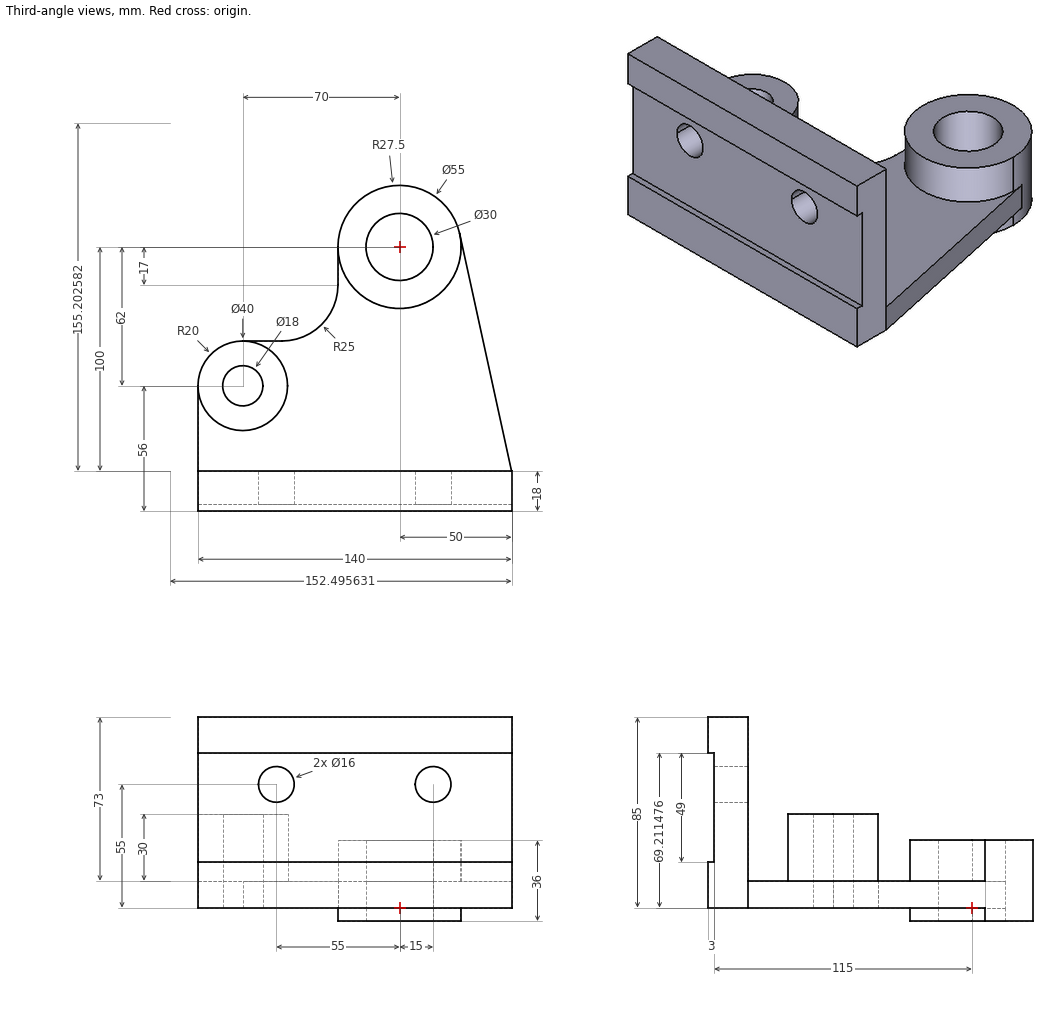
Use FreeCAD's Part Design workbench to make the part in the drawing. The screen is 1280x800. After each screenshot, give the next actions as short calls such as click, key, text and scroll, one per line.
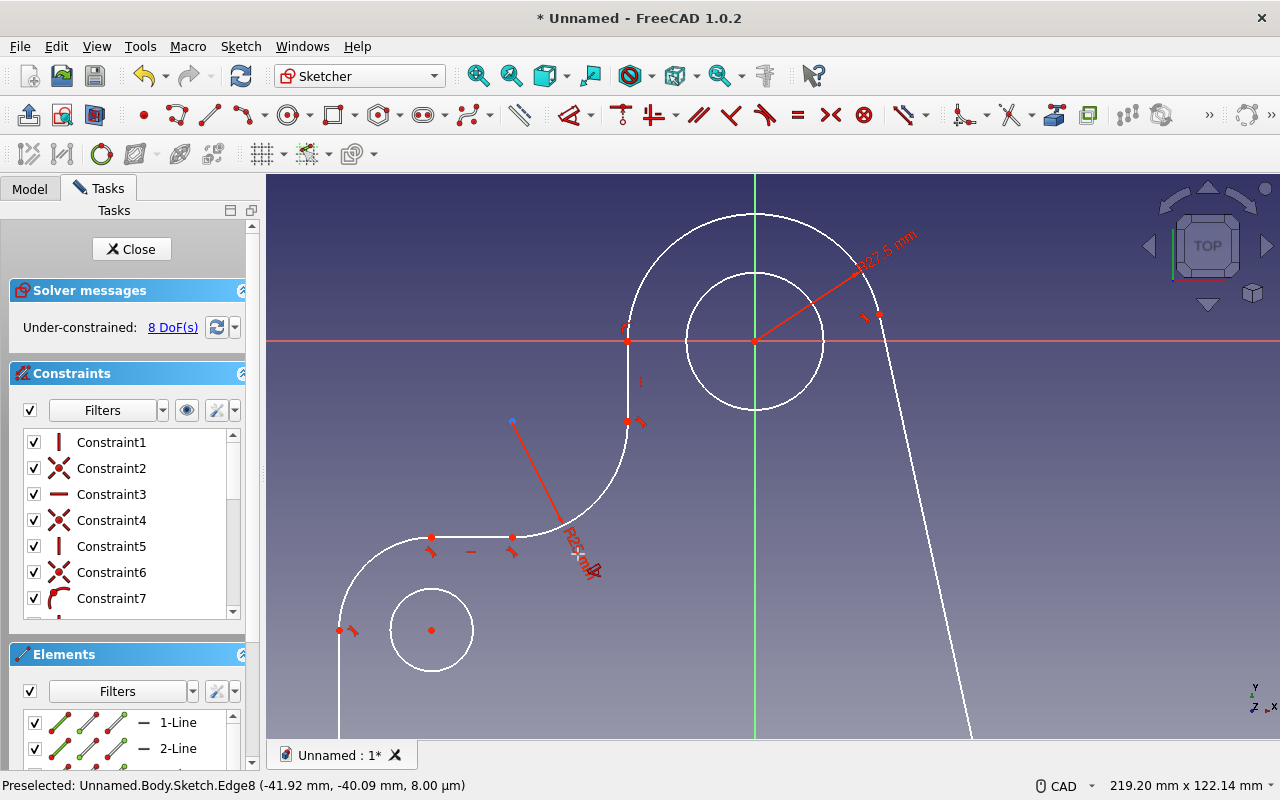
click(390, 548)
click(376, 519)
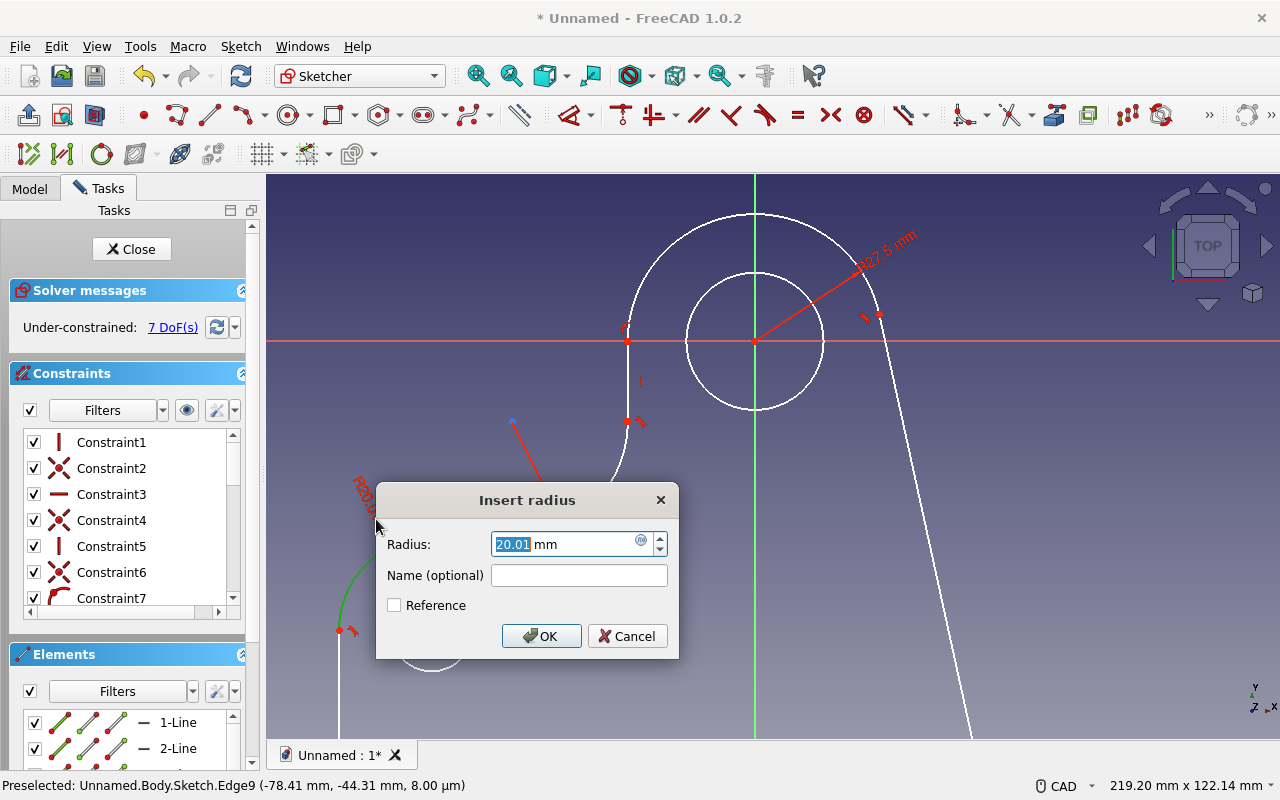
text(20)
key(Return)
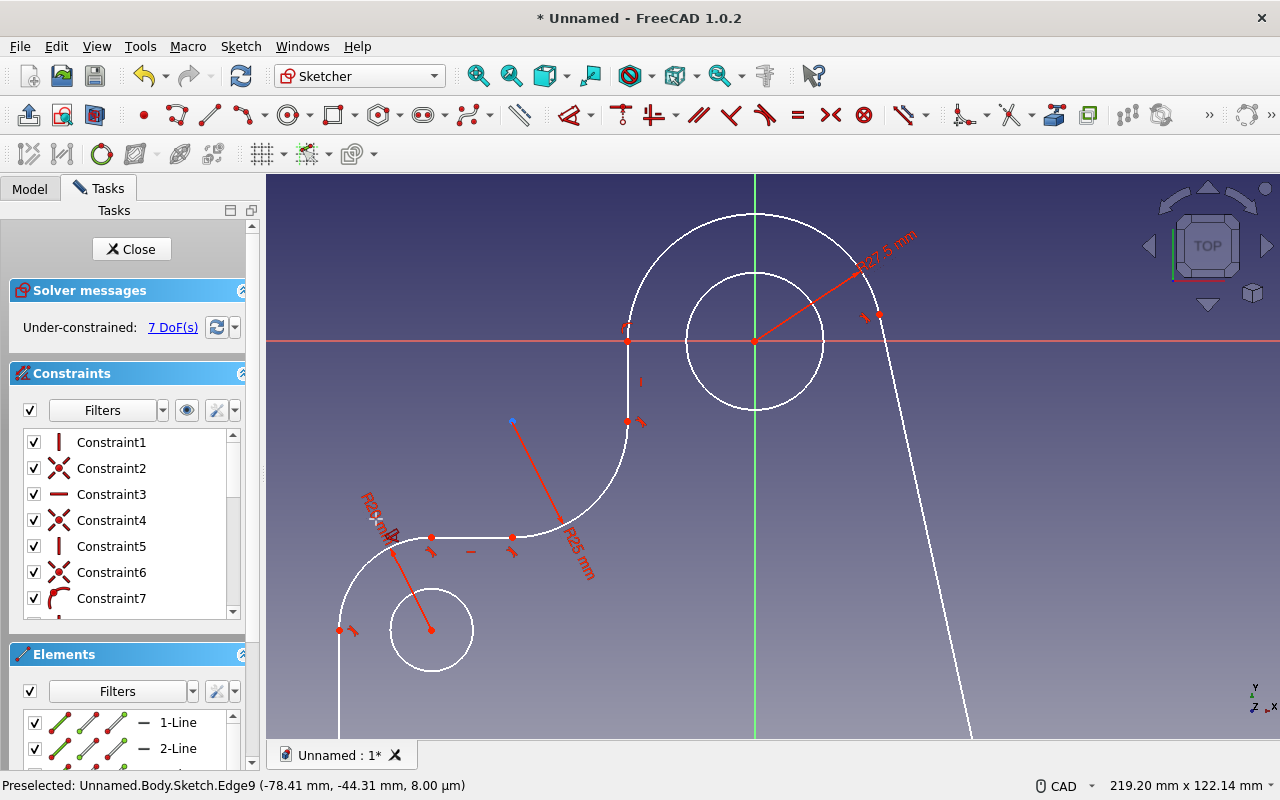
click(461, 601)
click(484, 578)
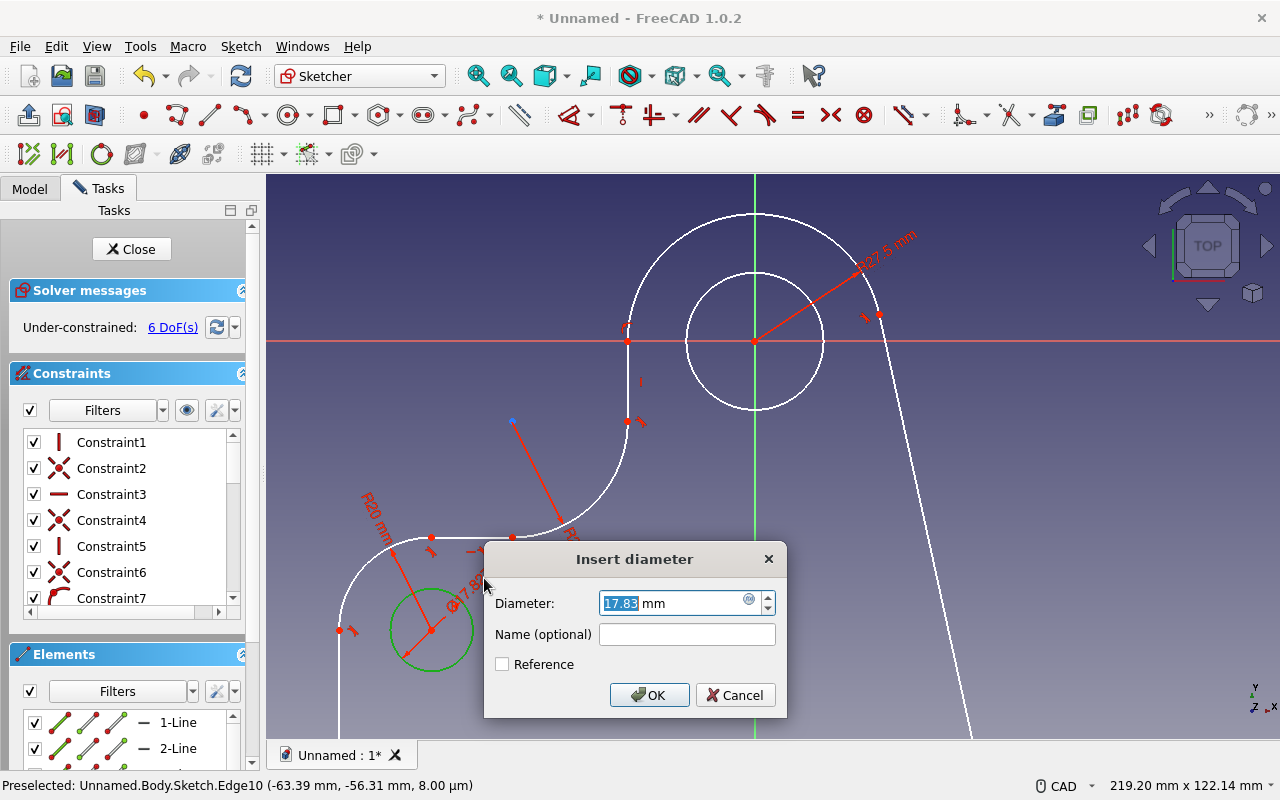
text(18)
key(Return)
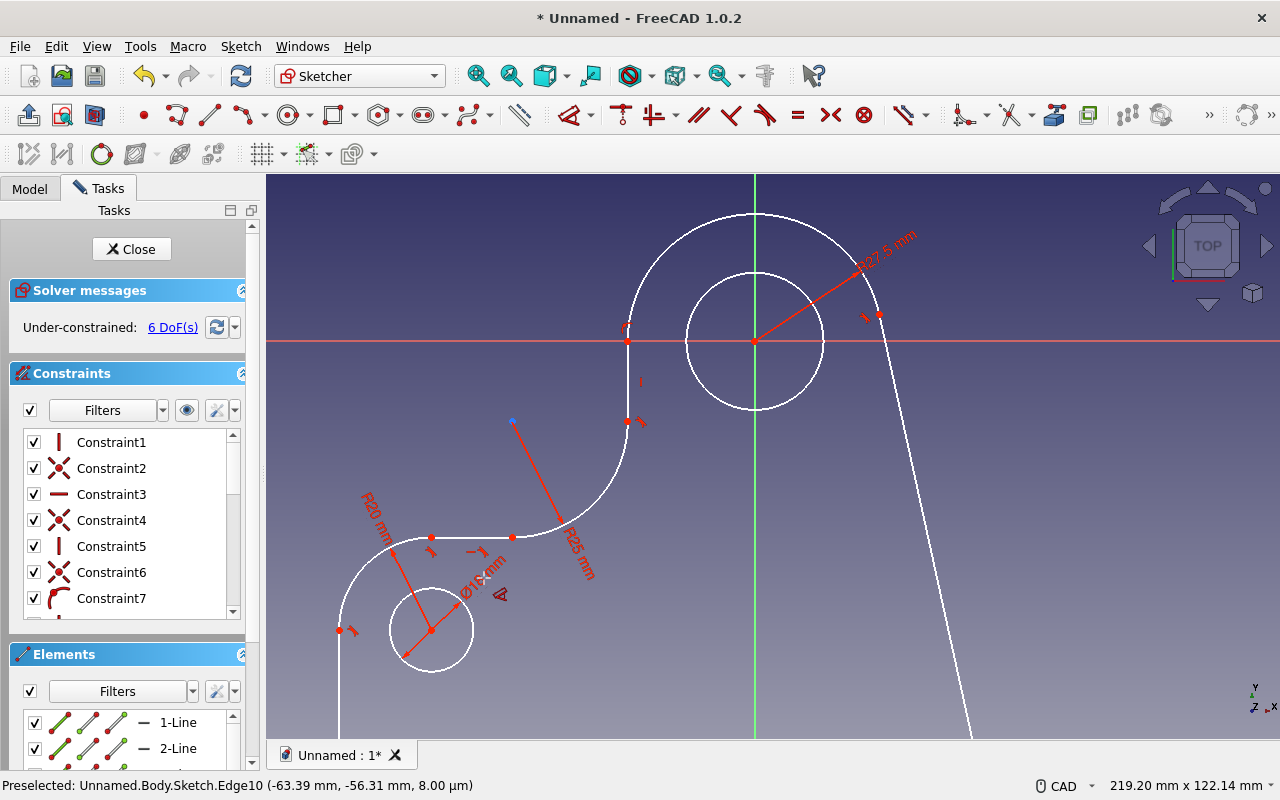
click(803, 293)
click(851, 313)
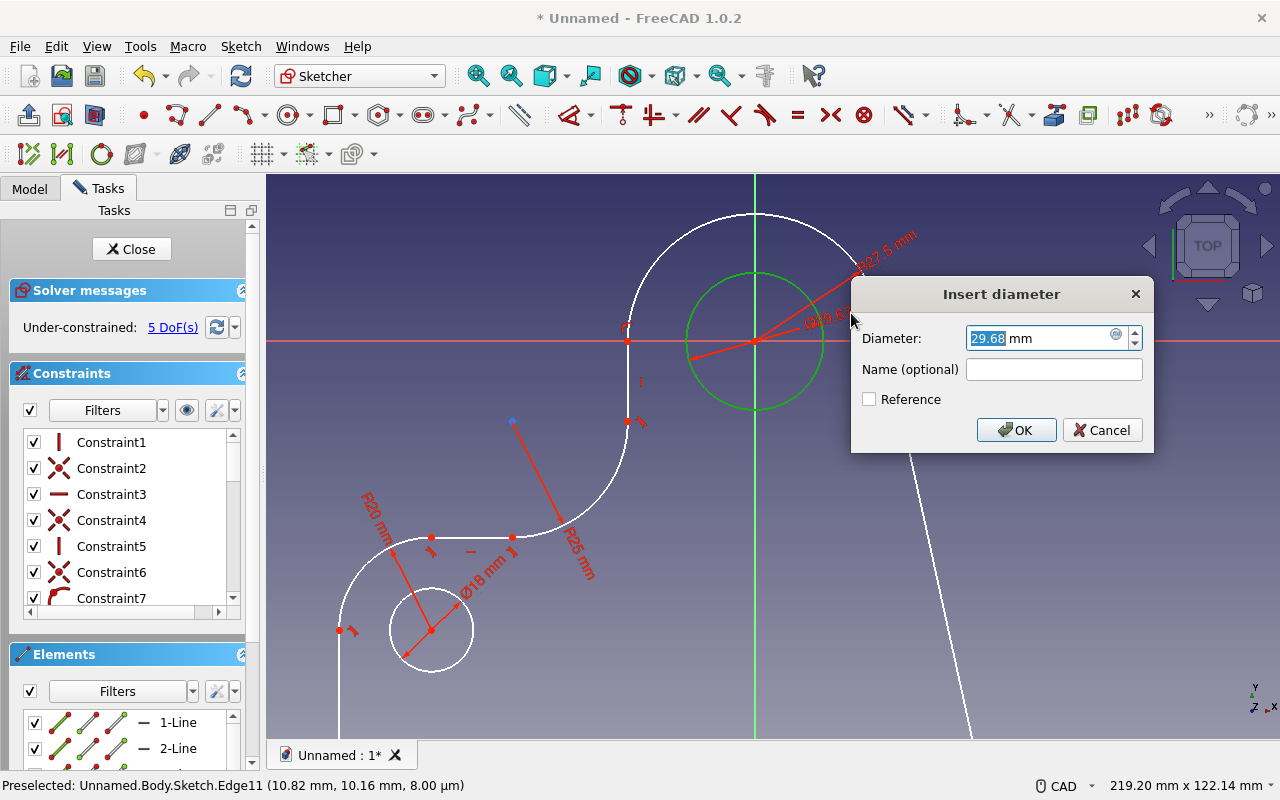
text(30)
key(Return)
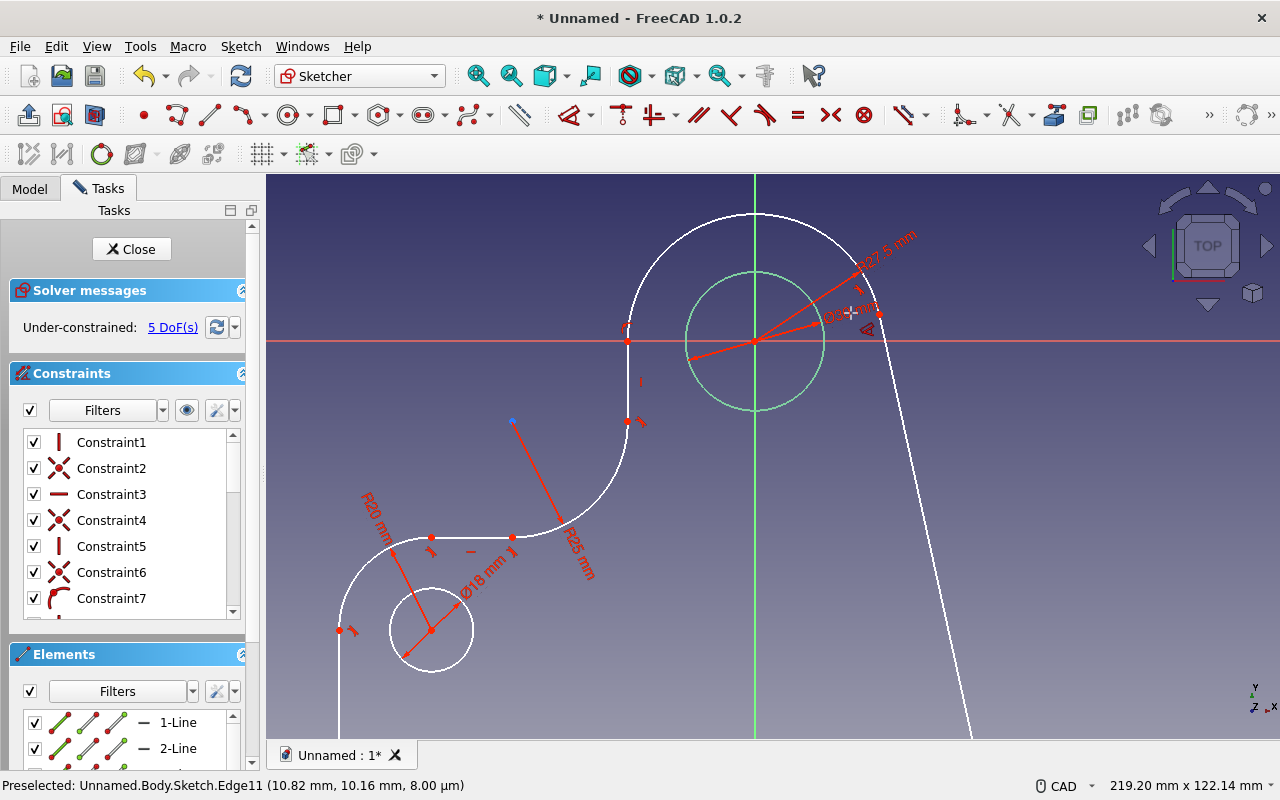
click(339, 708)
click(305, 671)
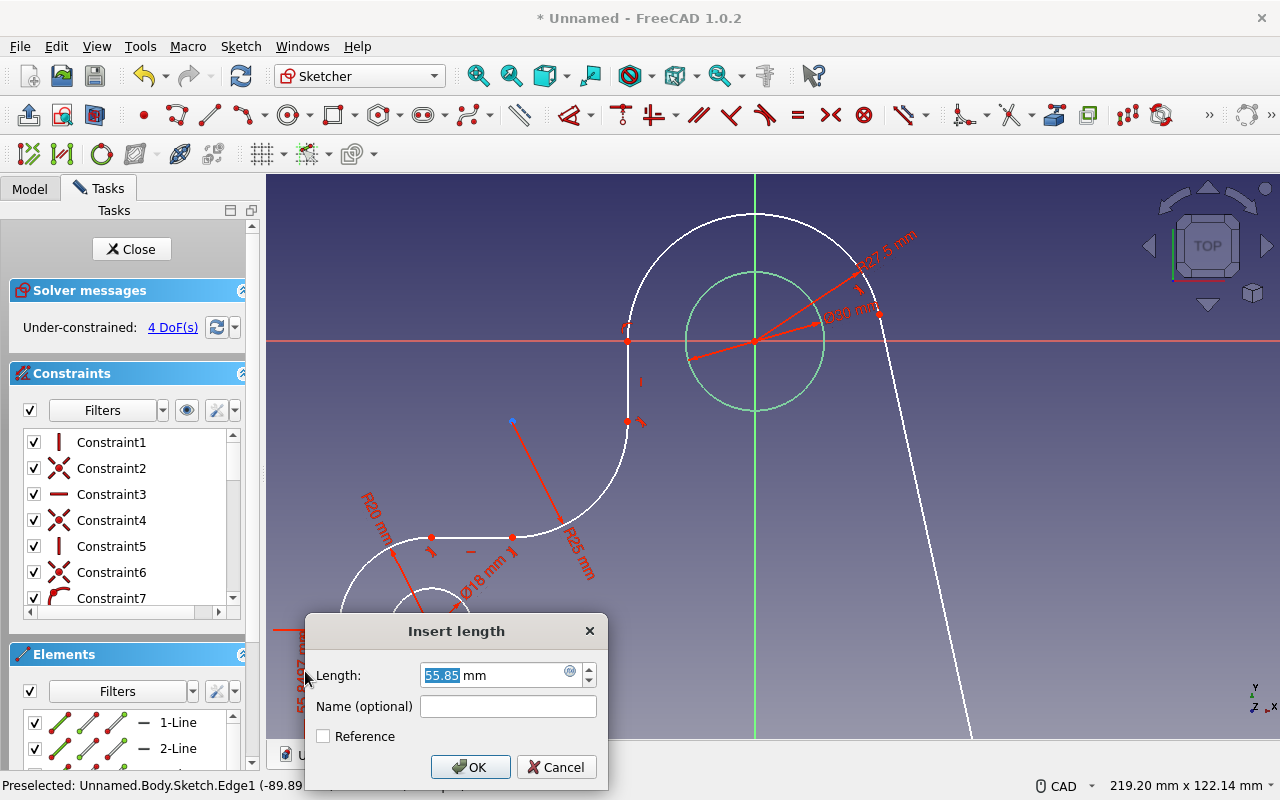
text(56)
key(Return)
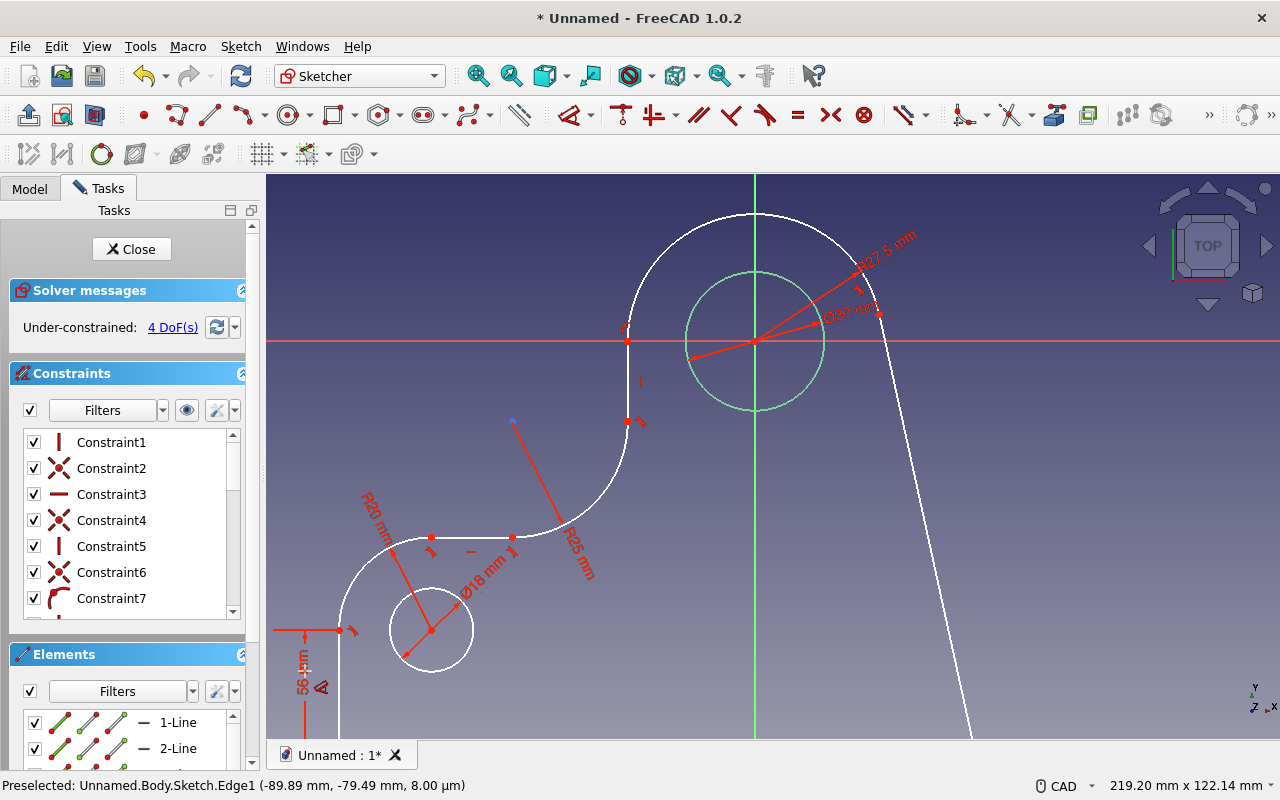
scroll(756, 342, down, 3)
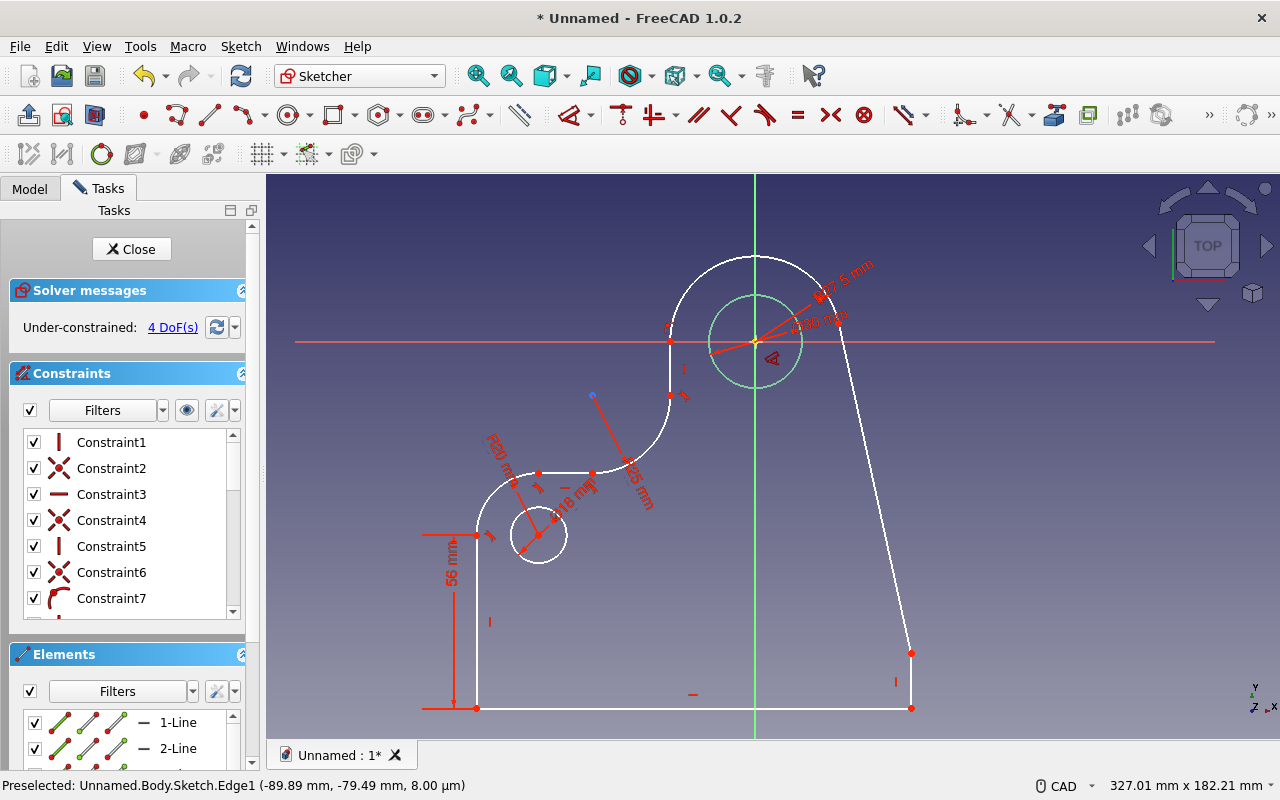
click(883, 629)
click(917, 620)